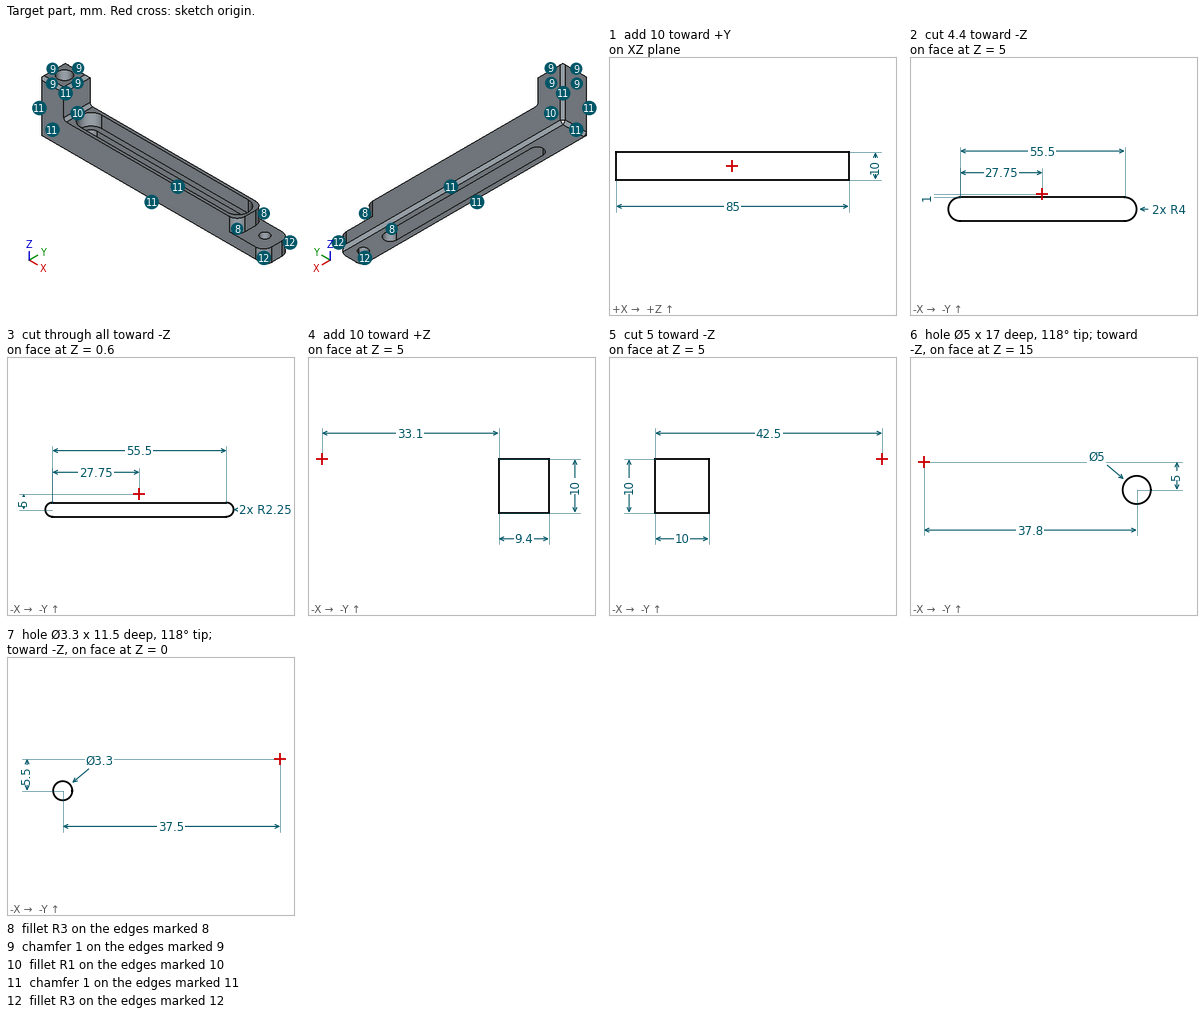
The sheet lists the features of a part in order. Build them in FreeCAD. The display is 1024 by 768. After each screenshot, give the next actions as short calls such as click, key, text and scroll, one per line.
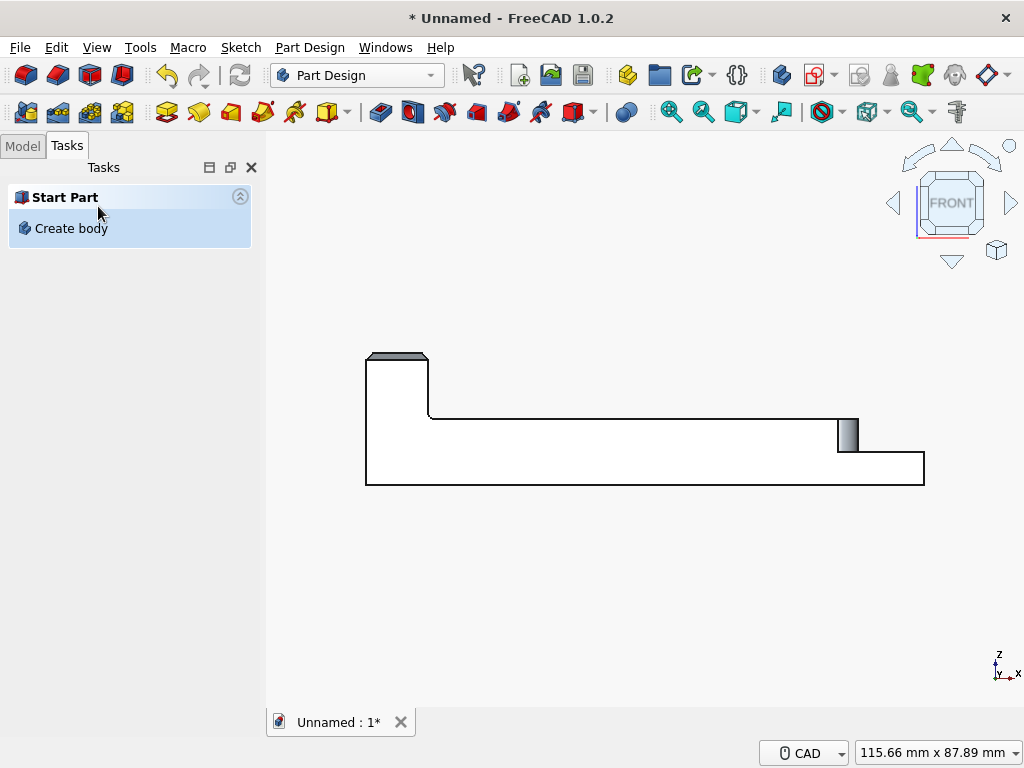
click(366, 434)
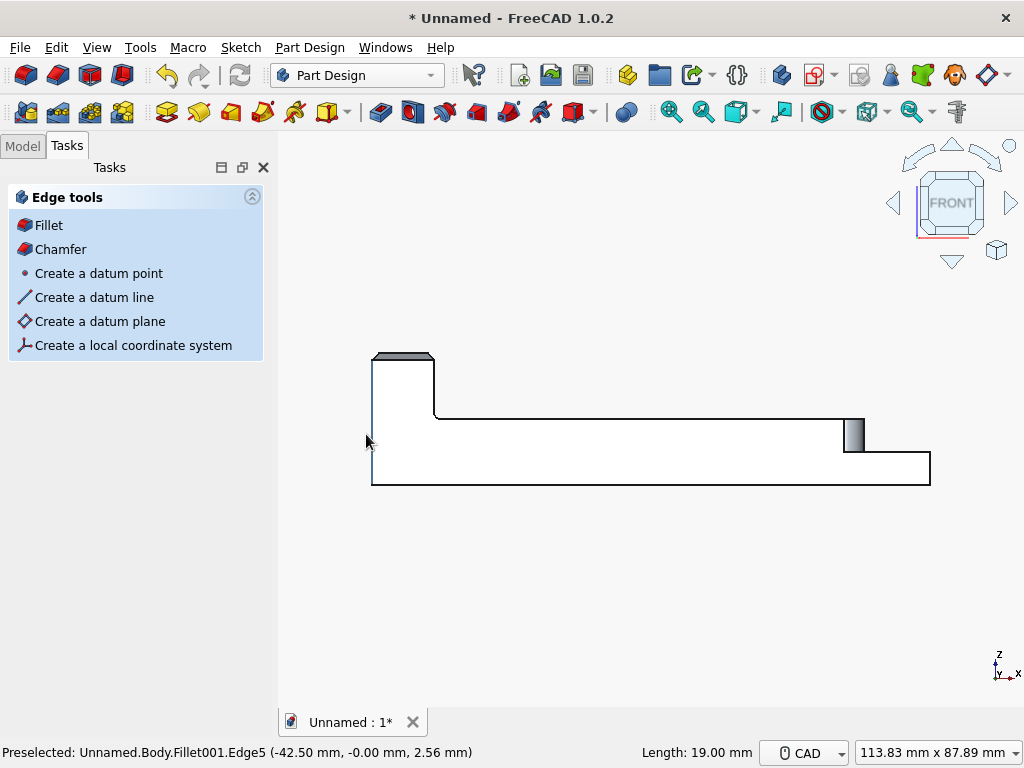
key(3)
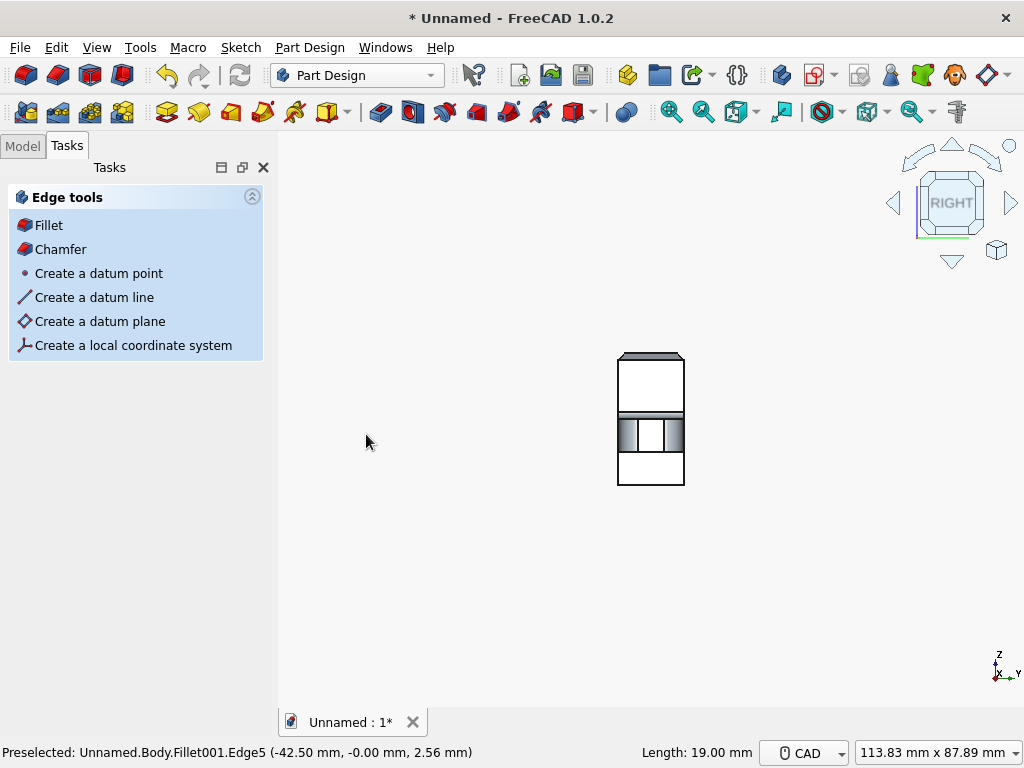
click(672, 112)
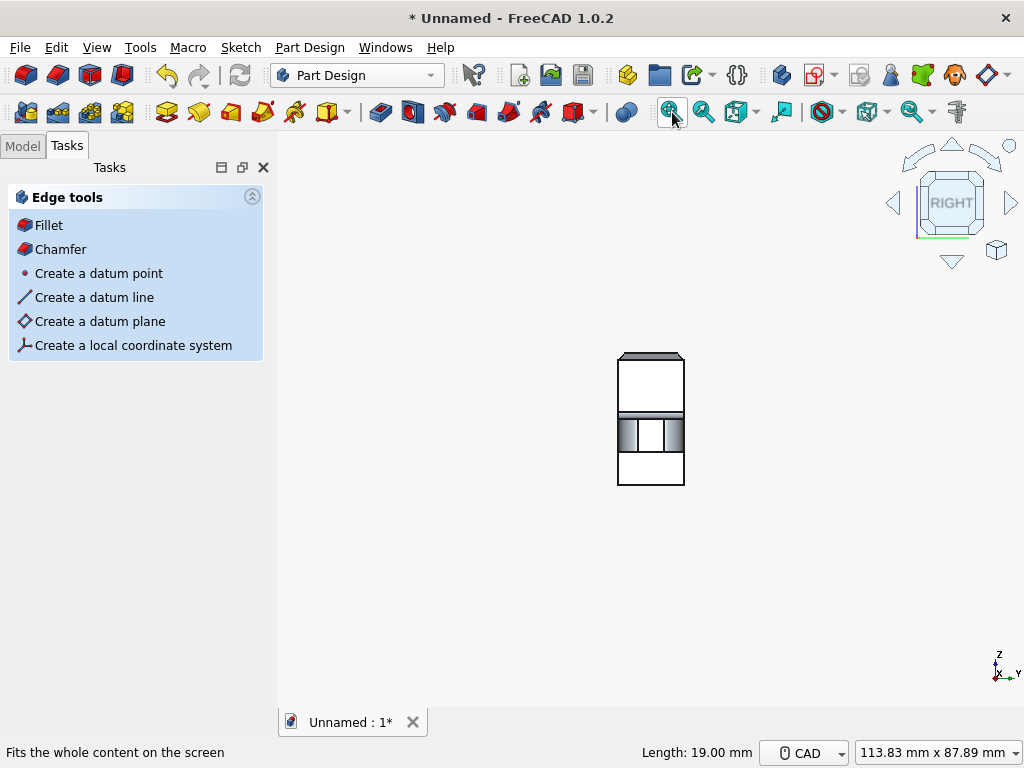
key(5)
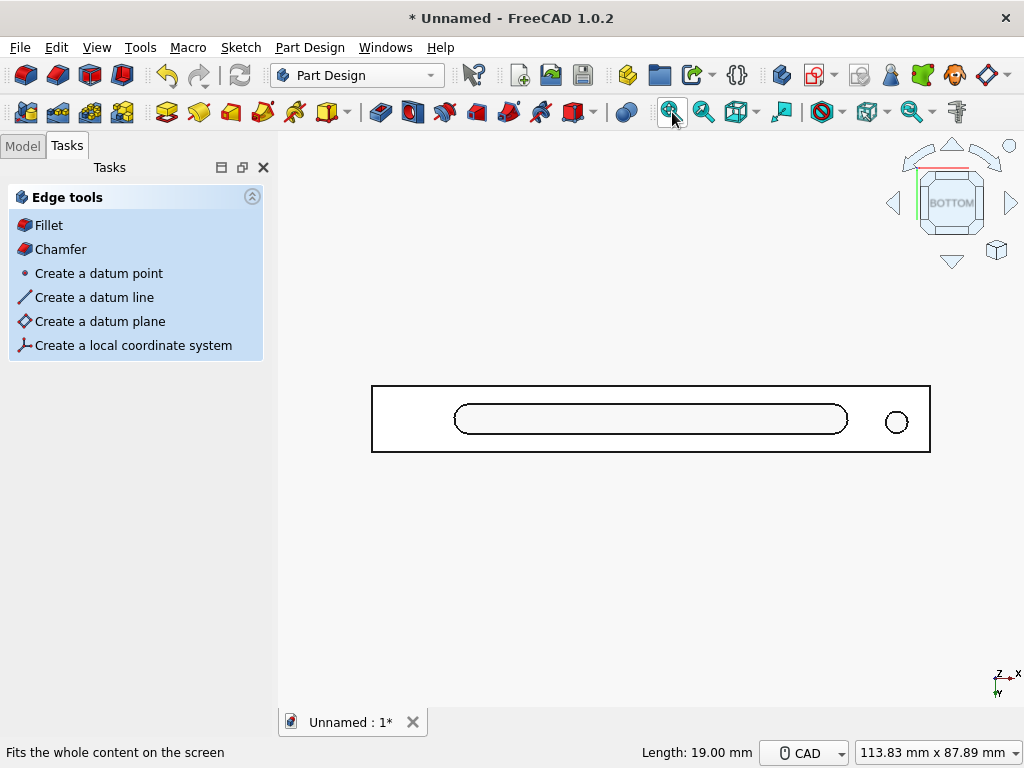
click(651, 385, ctrl)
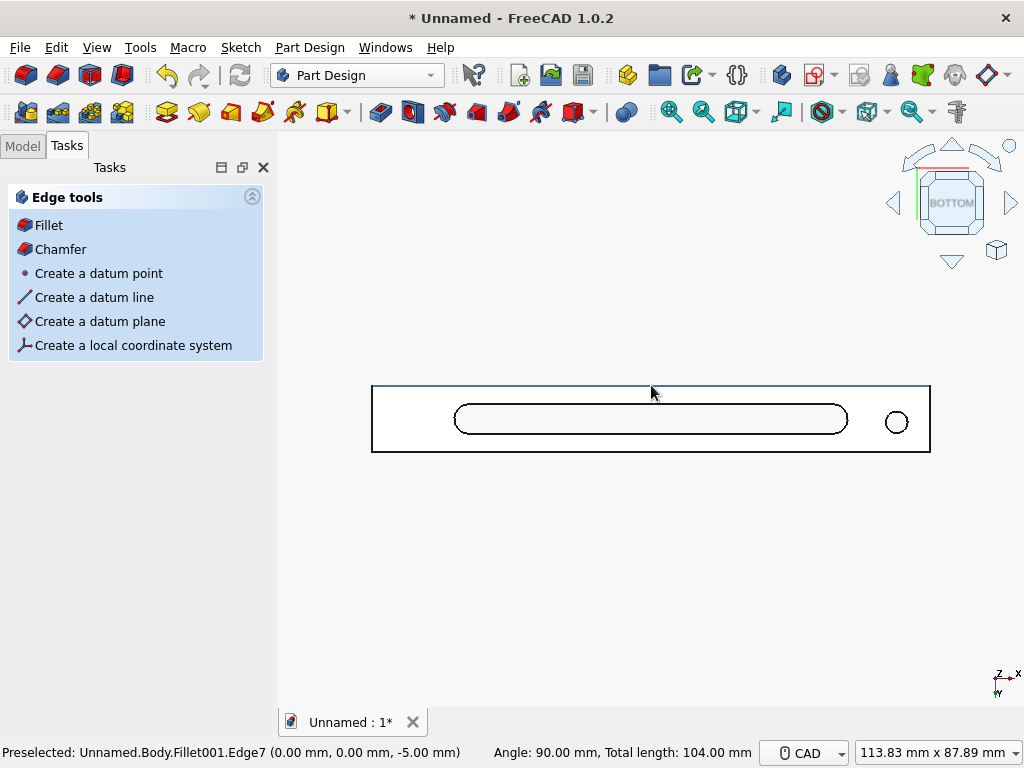
click(372, 418, ctrl)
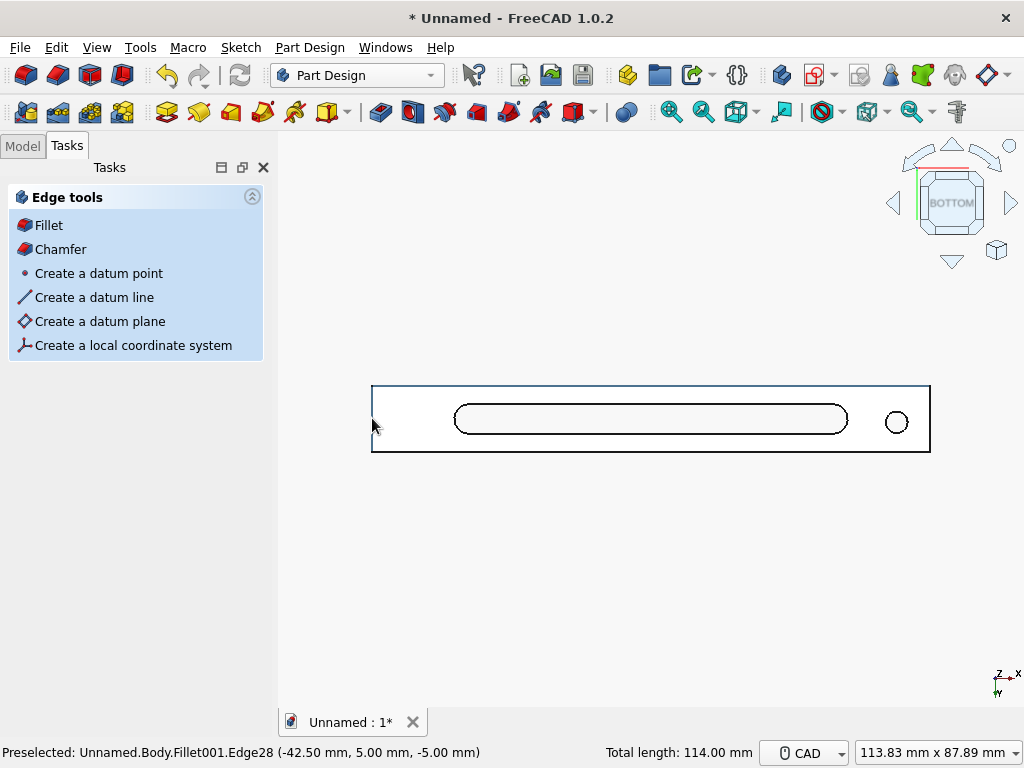
key(4)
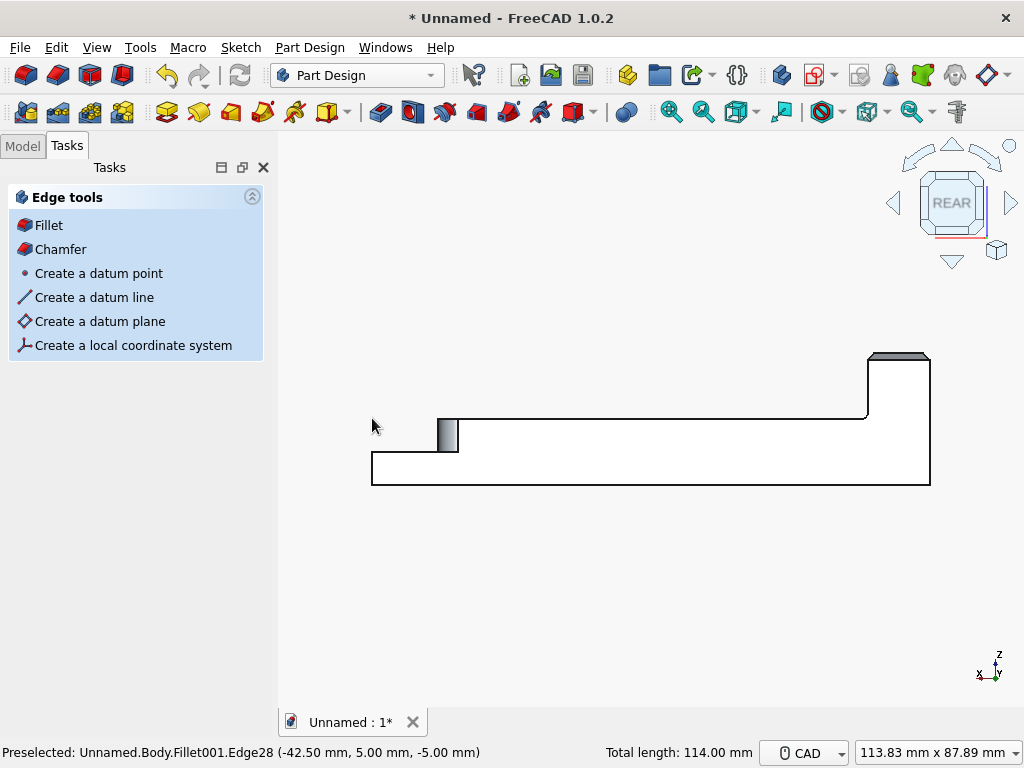
click(651, 484, ctrl)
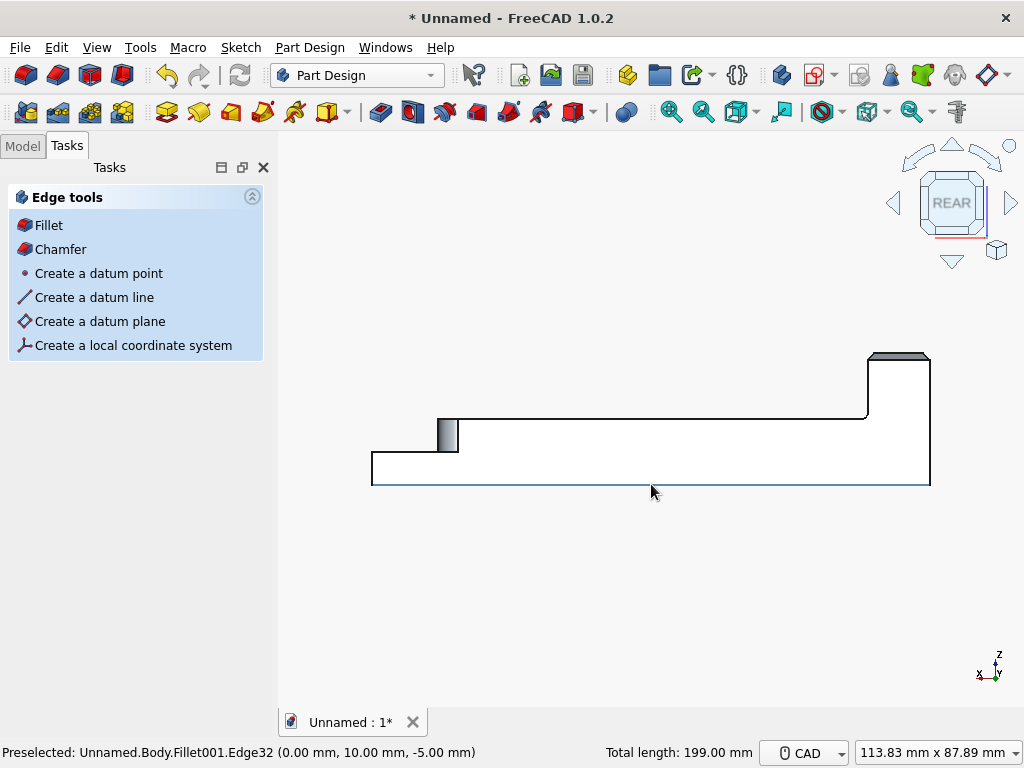
click(930, 421, ctrl)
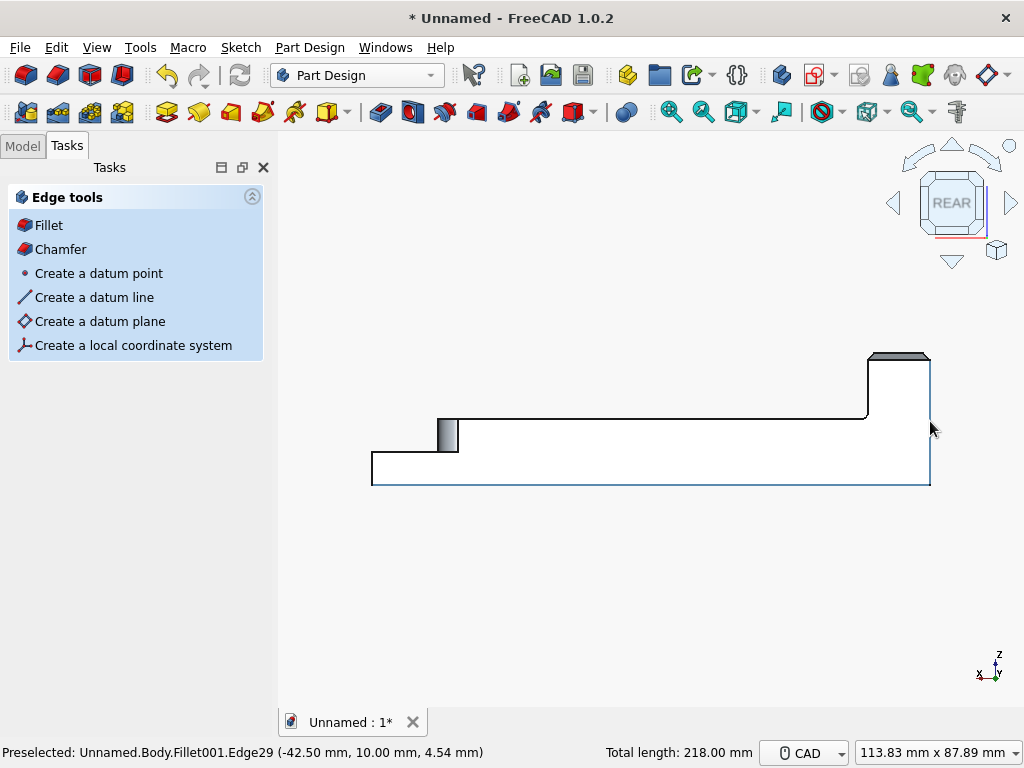
click(58, 76)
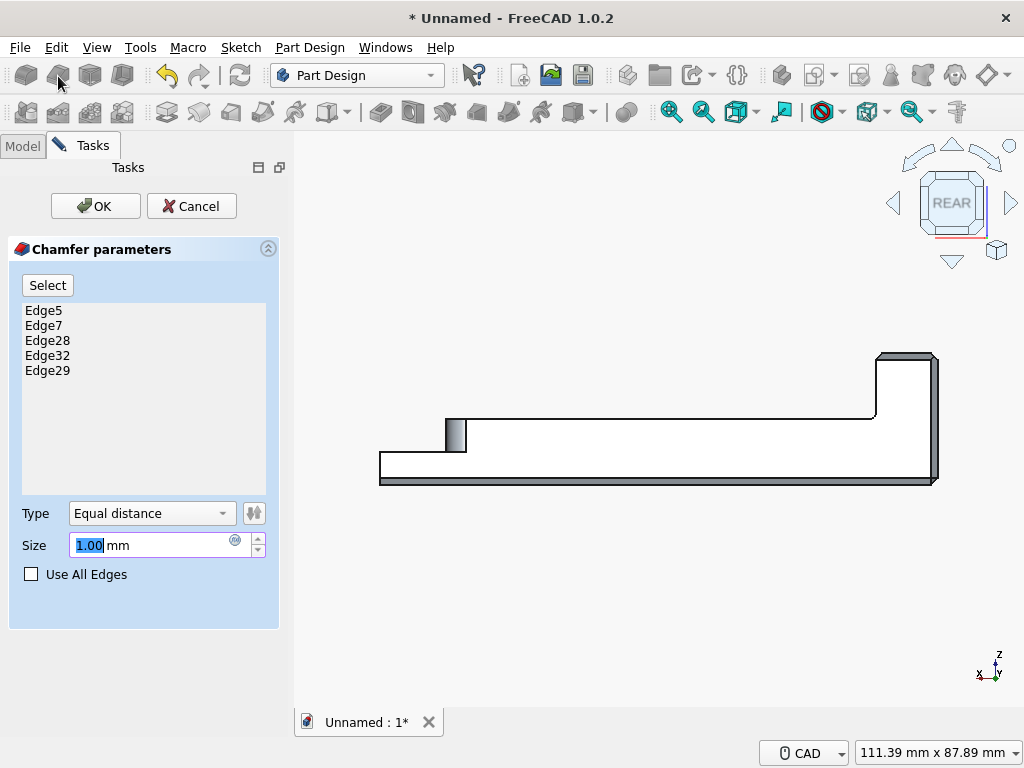
text(1)
key(Tab)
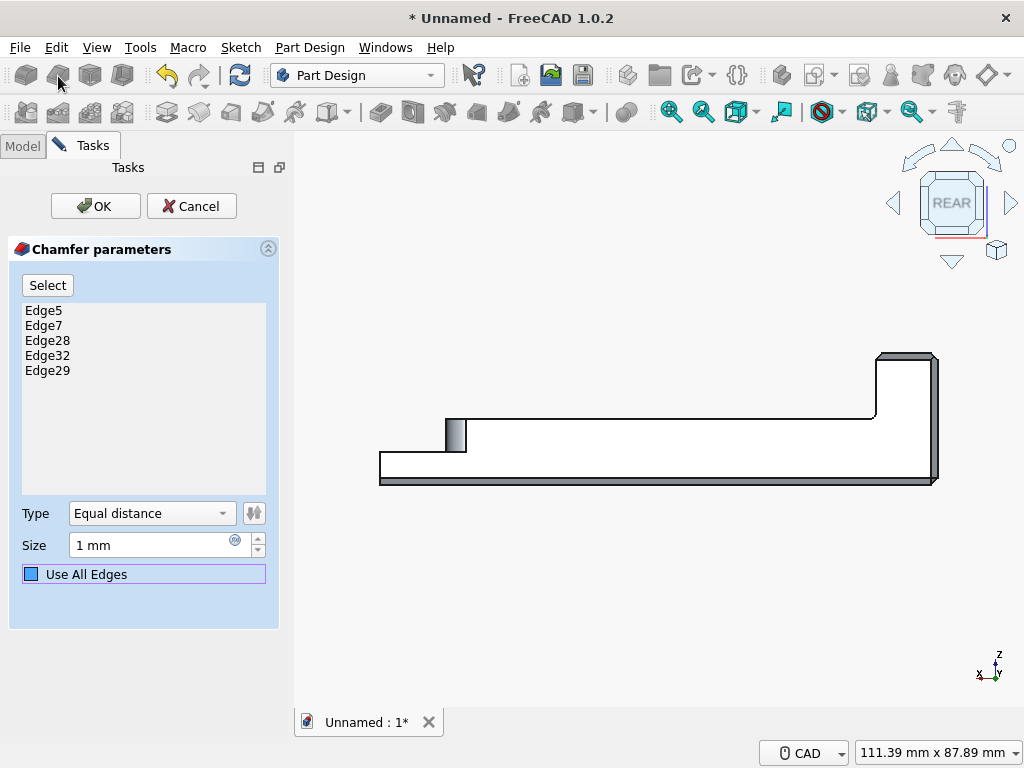
click(96, 206)